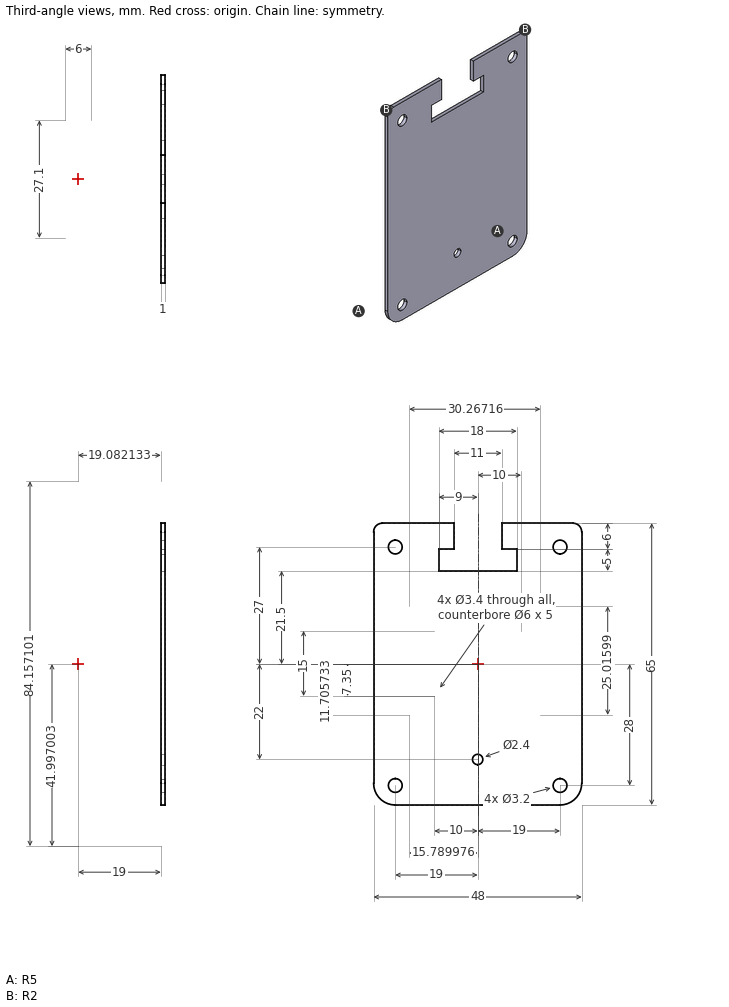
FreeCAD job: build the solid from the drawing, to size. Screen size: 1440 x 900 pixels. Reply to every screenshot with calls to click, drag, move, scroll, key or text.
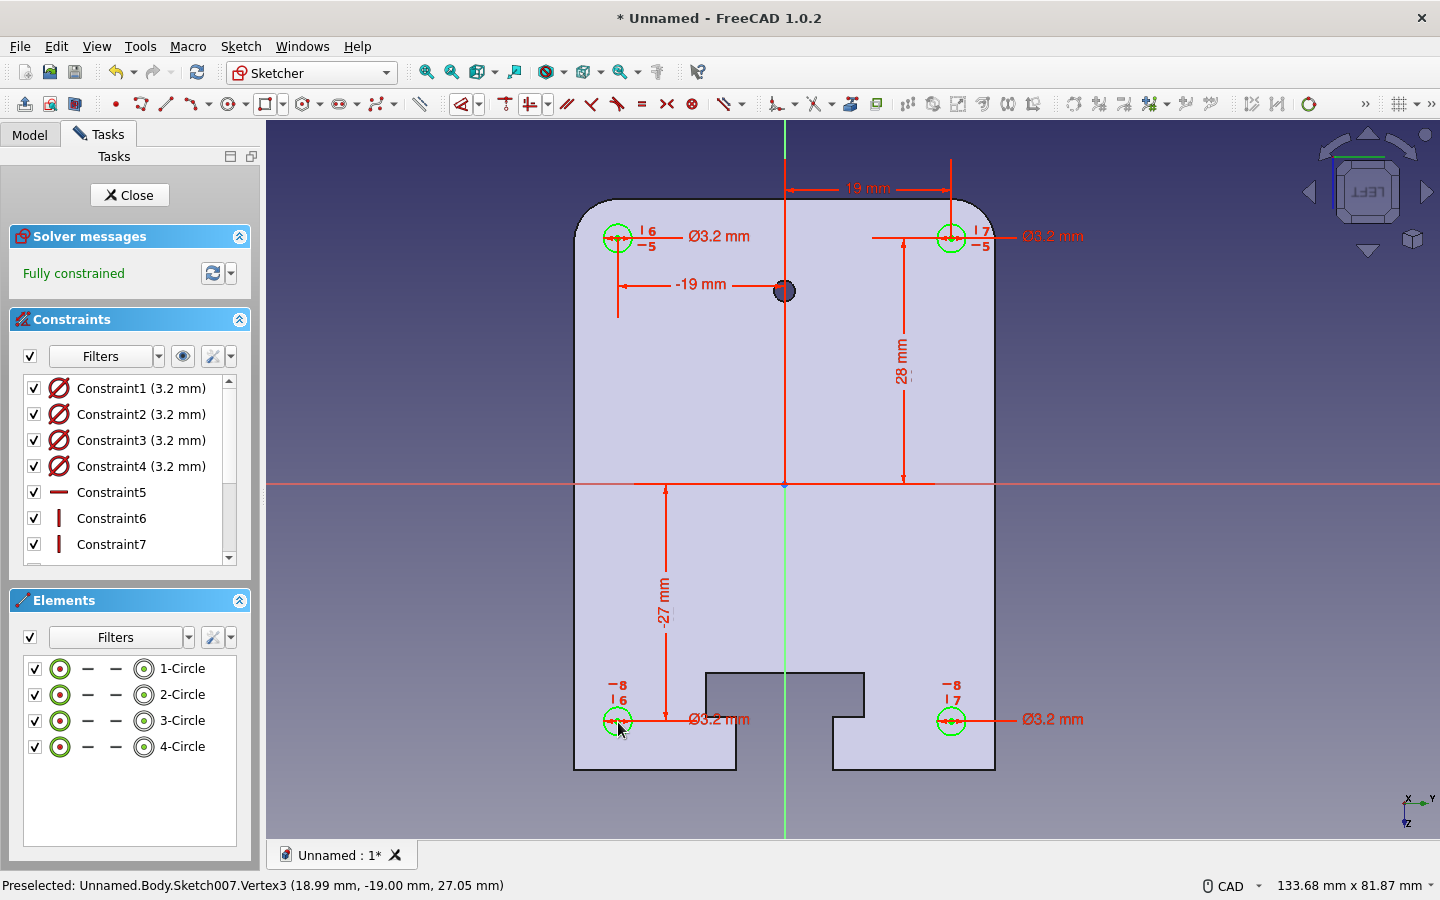
click(130, 195)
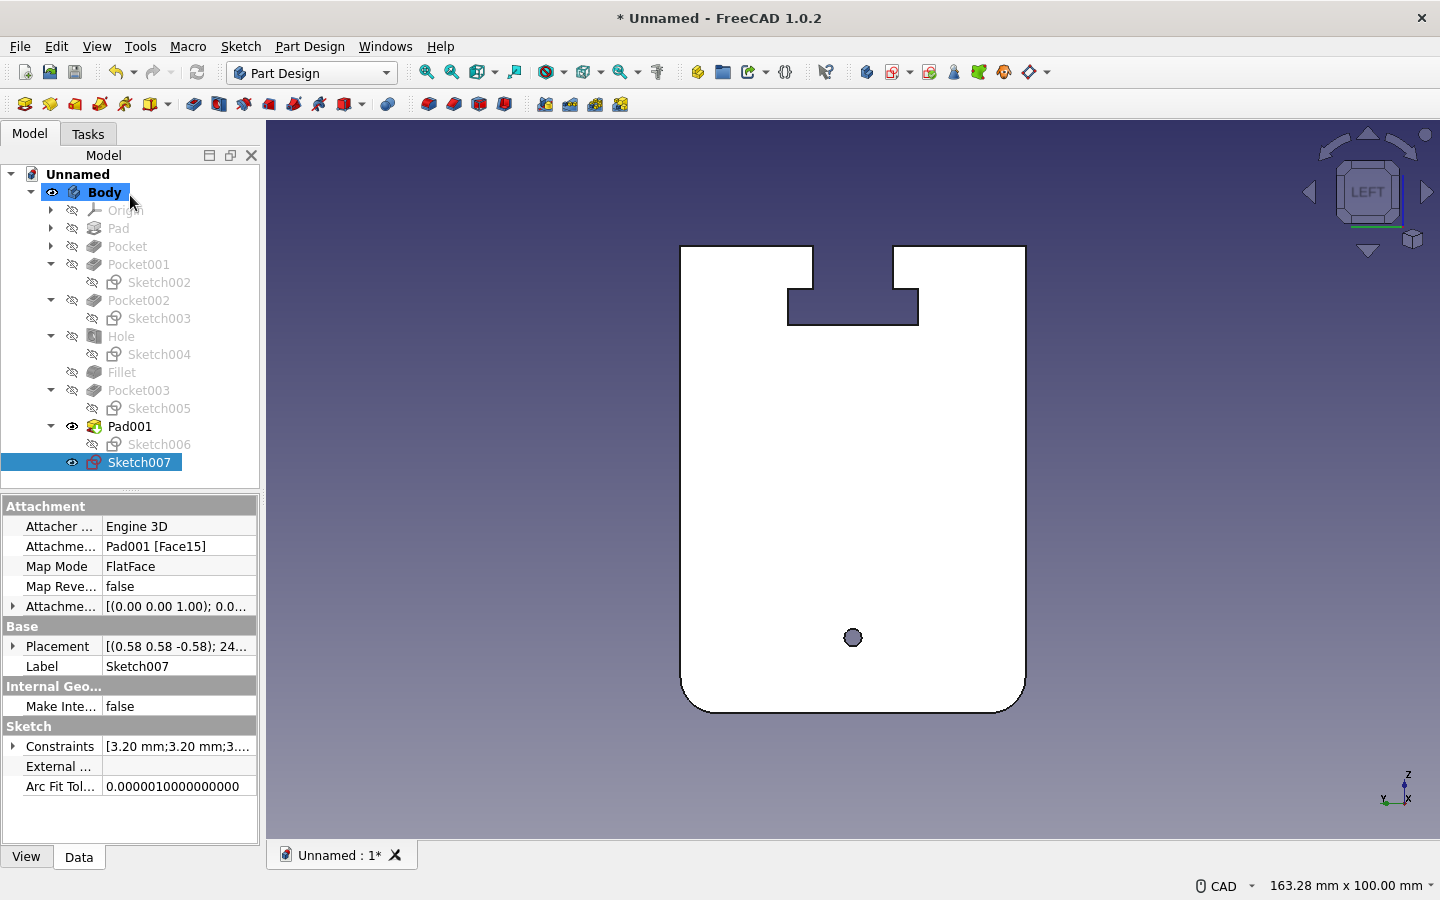
click(194, 104)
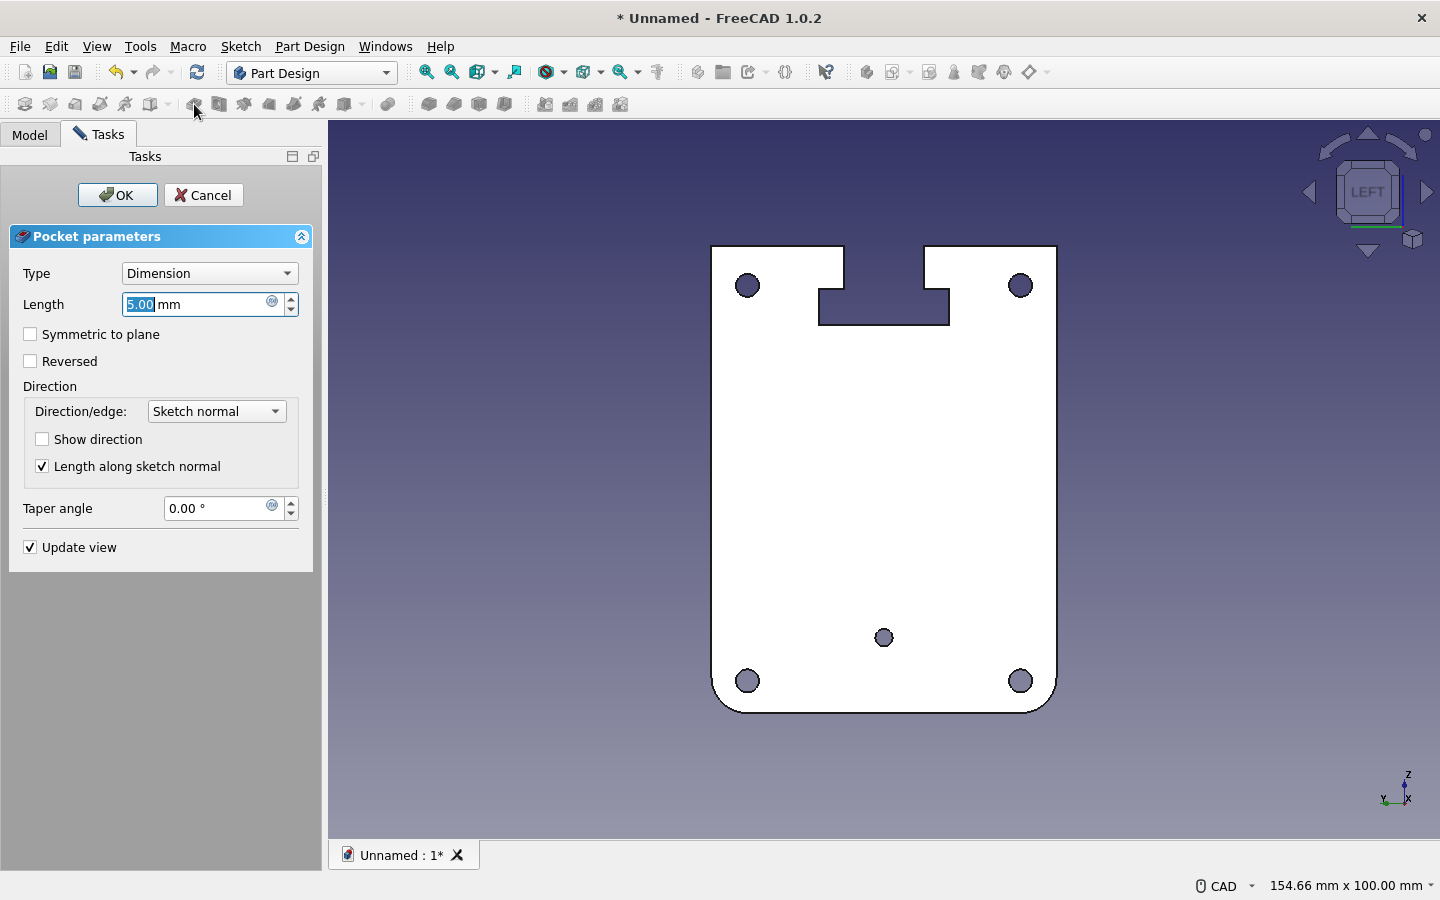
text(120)
key(Tab)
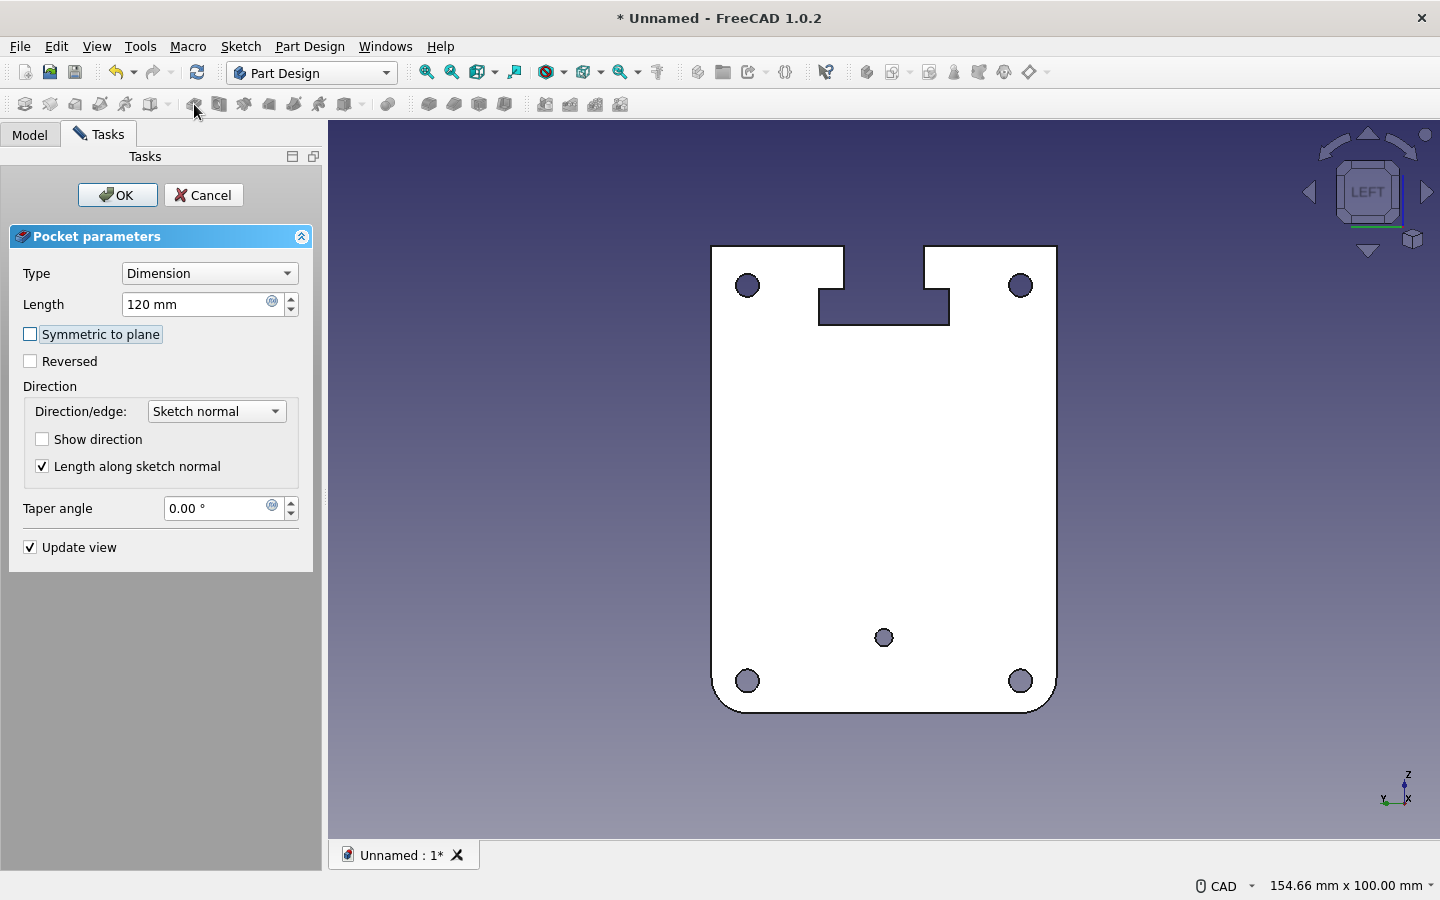
click(118, 195)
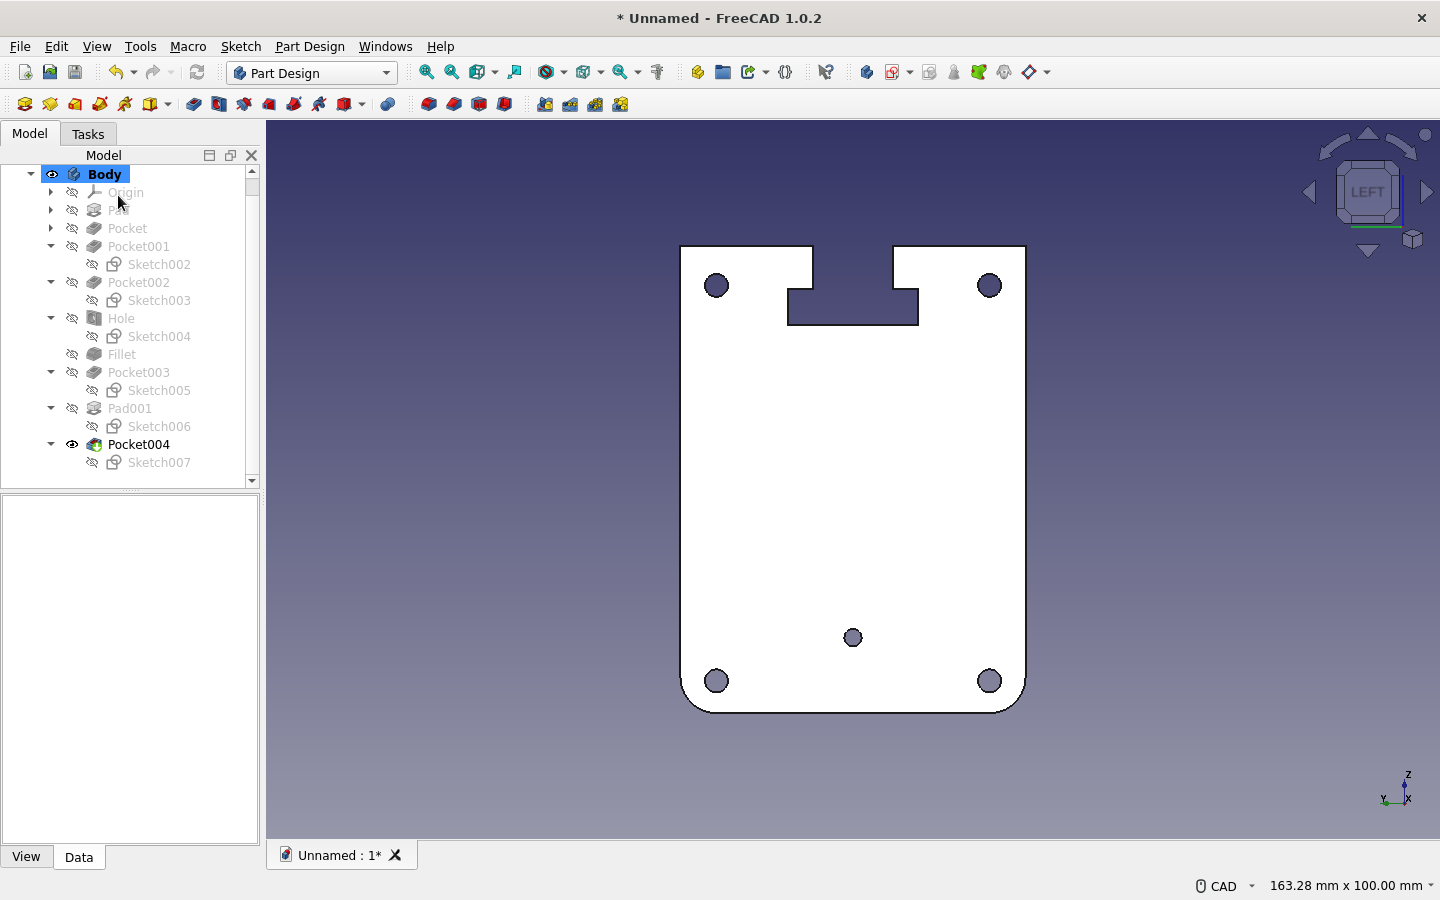
scroll(1026, 245, up, 9)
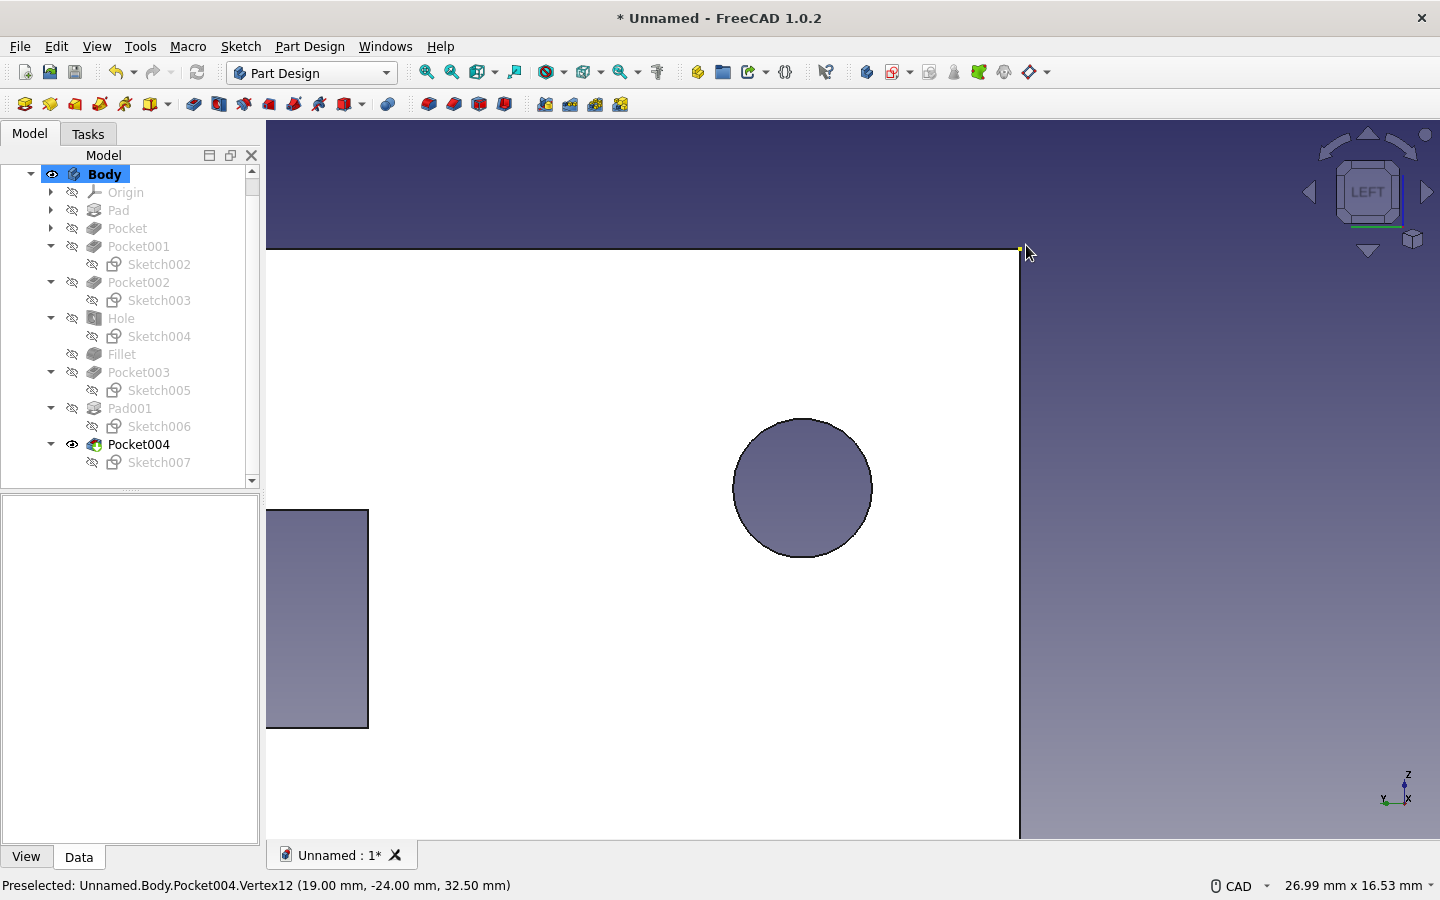
key(v)
key(f)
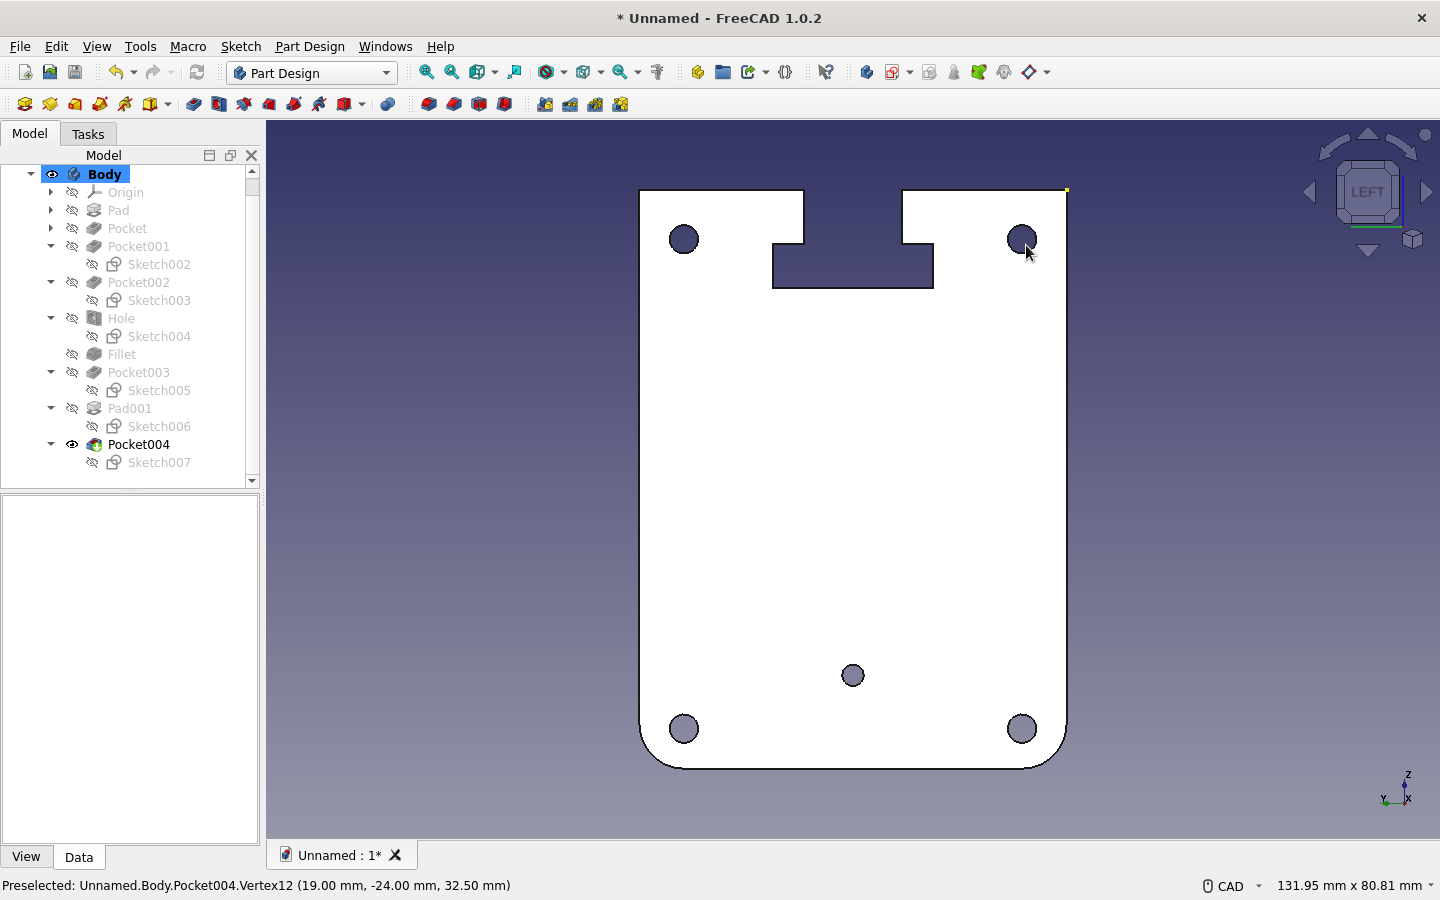
key(0)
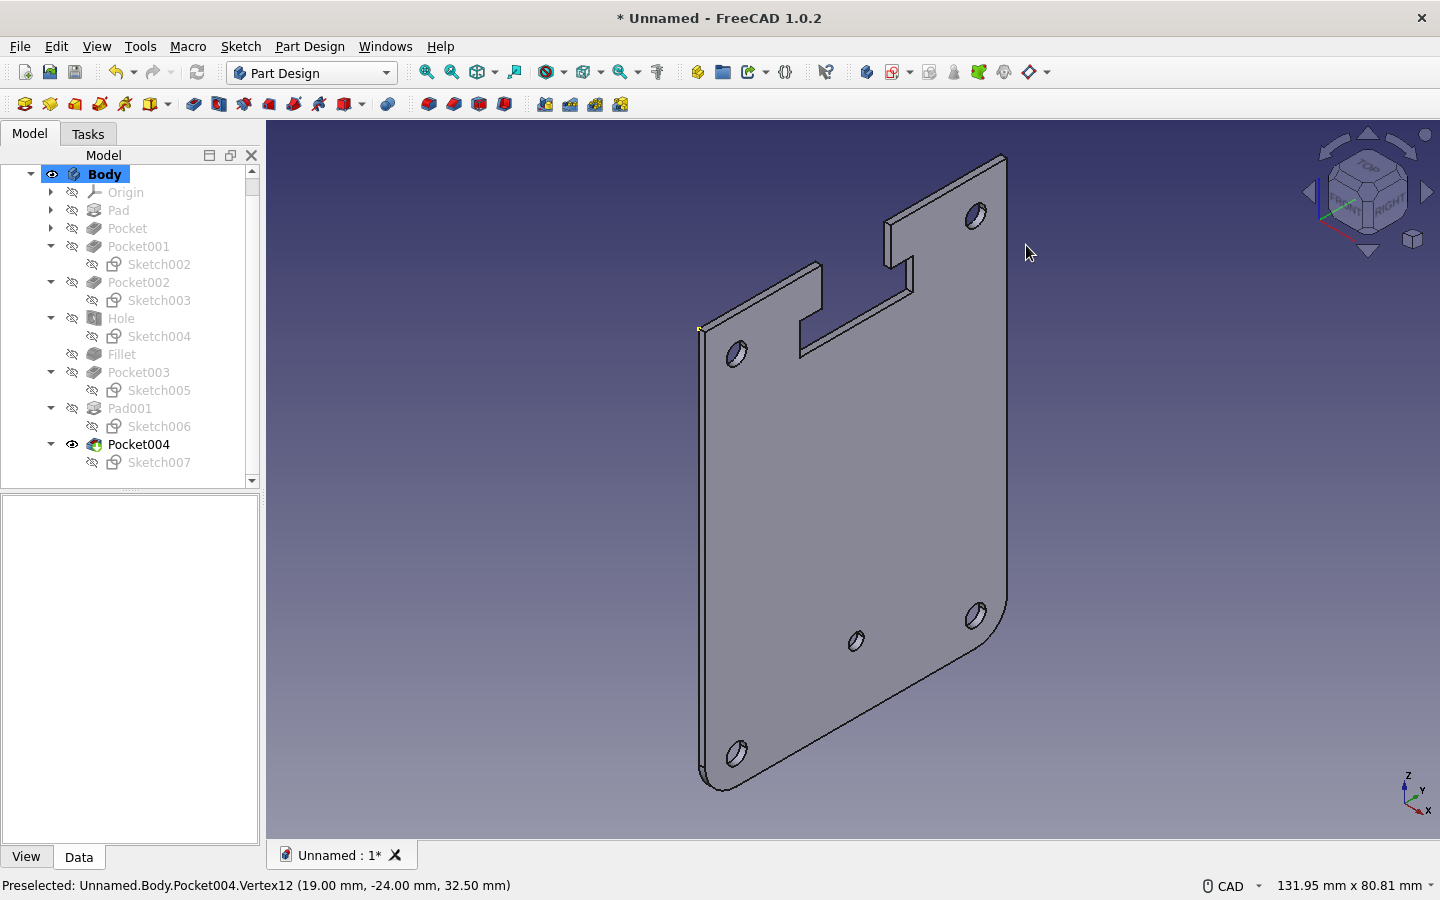
scroll(702, 330, up, 8)